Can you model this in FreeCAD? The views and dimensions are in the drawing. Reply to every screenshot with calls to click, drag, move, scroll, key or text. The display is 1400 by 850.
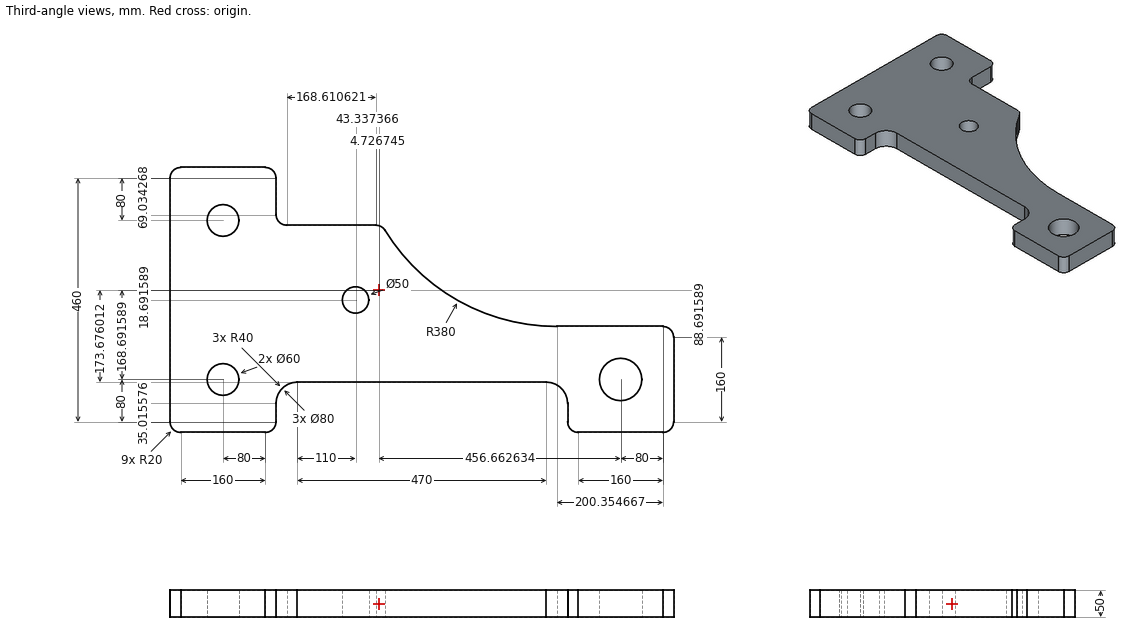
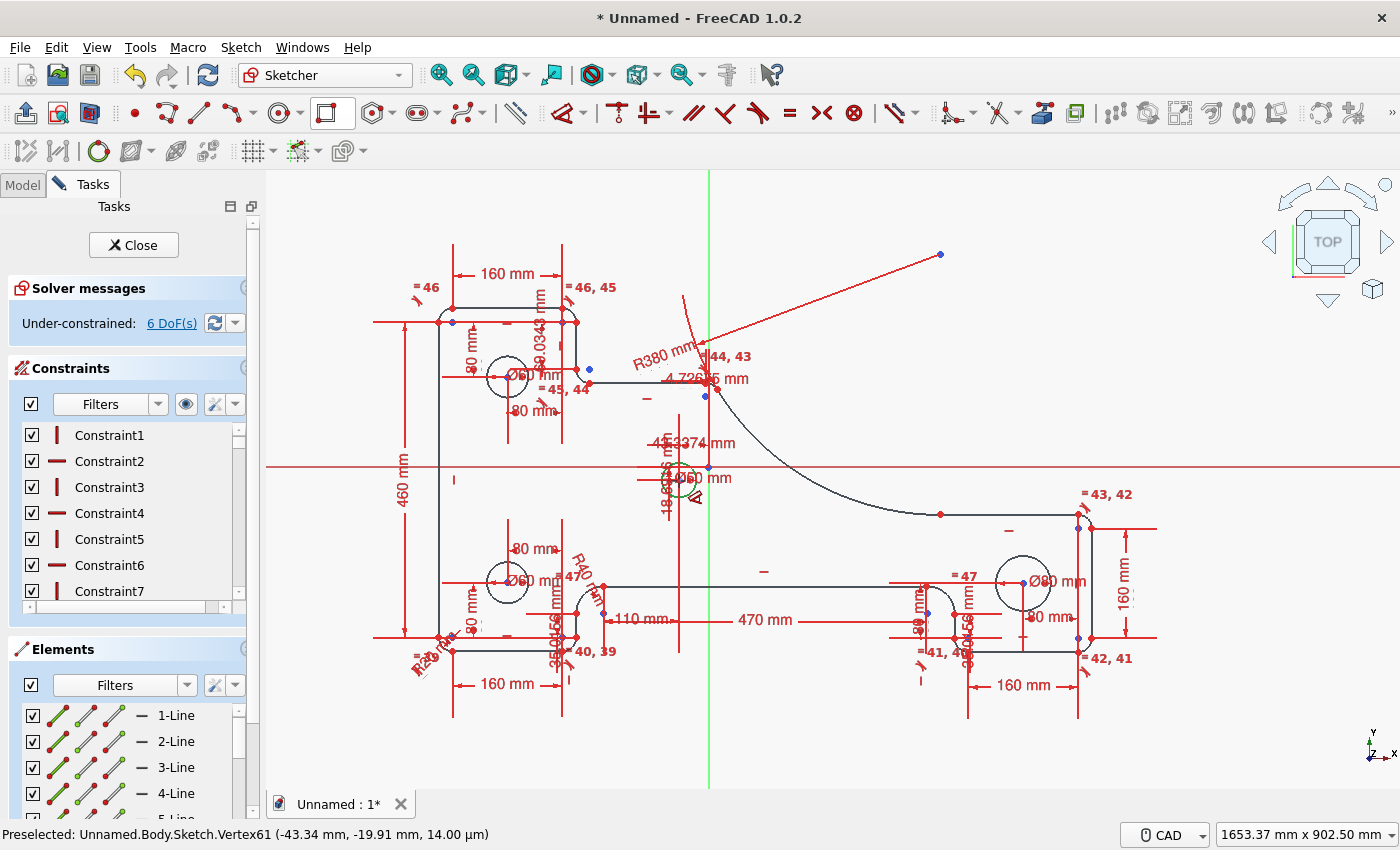
click(1037, 515)
click(977, 549)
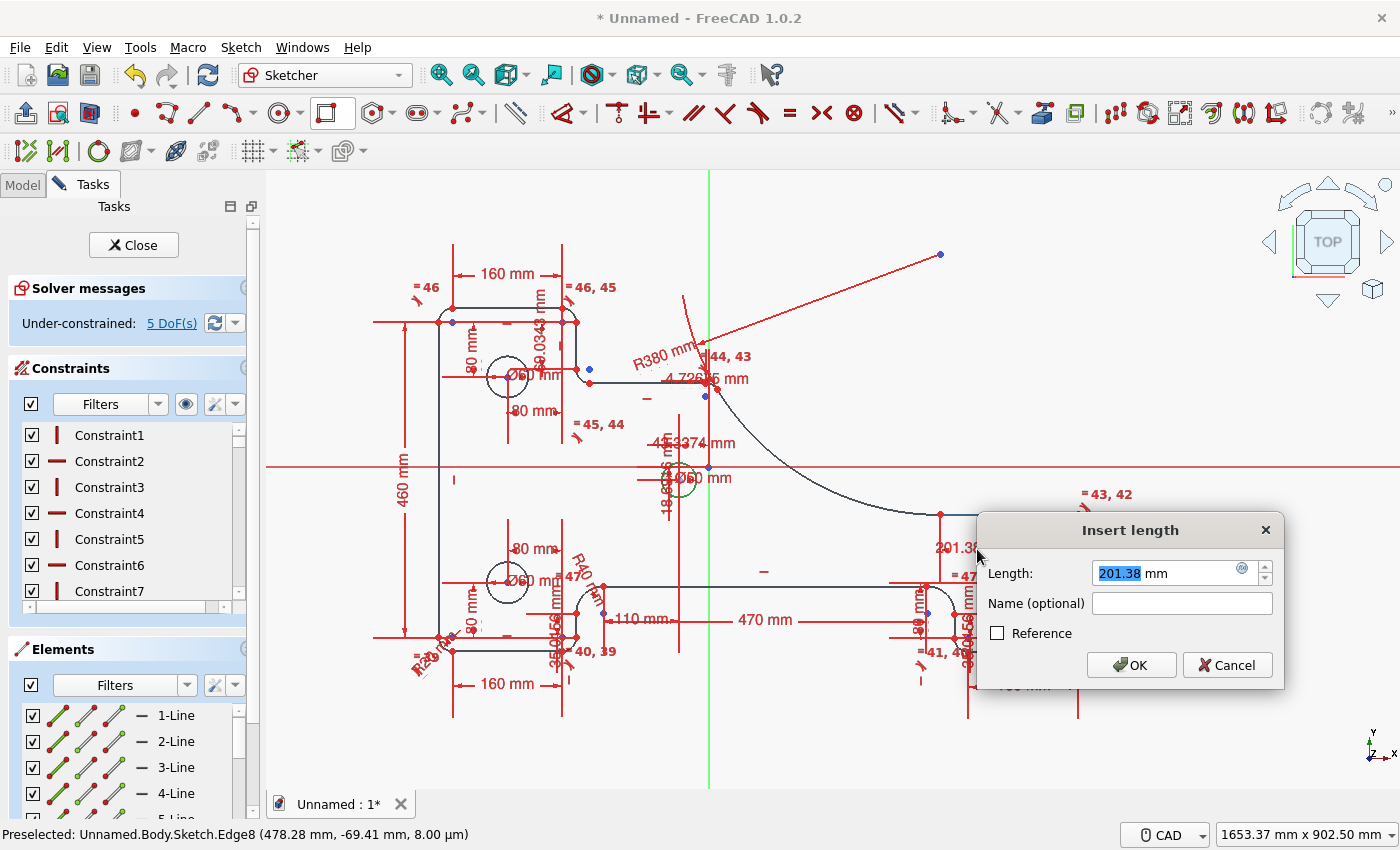
text(200.354667)
key(Return)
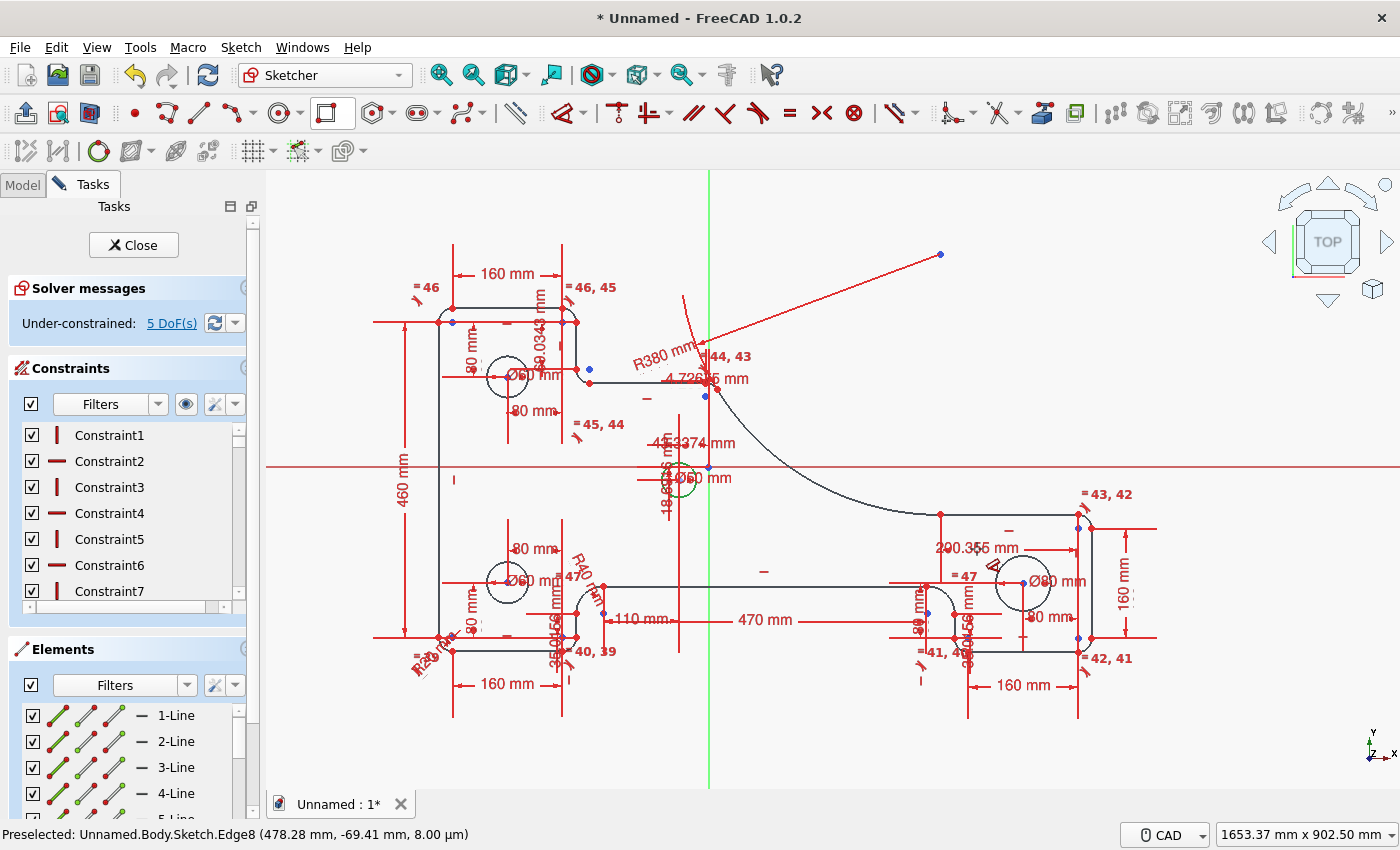
click(671, 383)
click(648, 417)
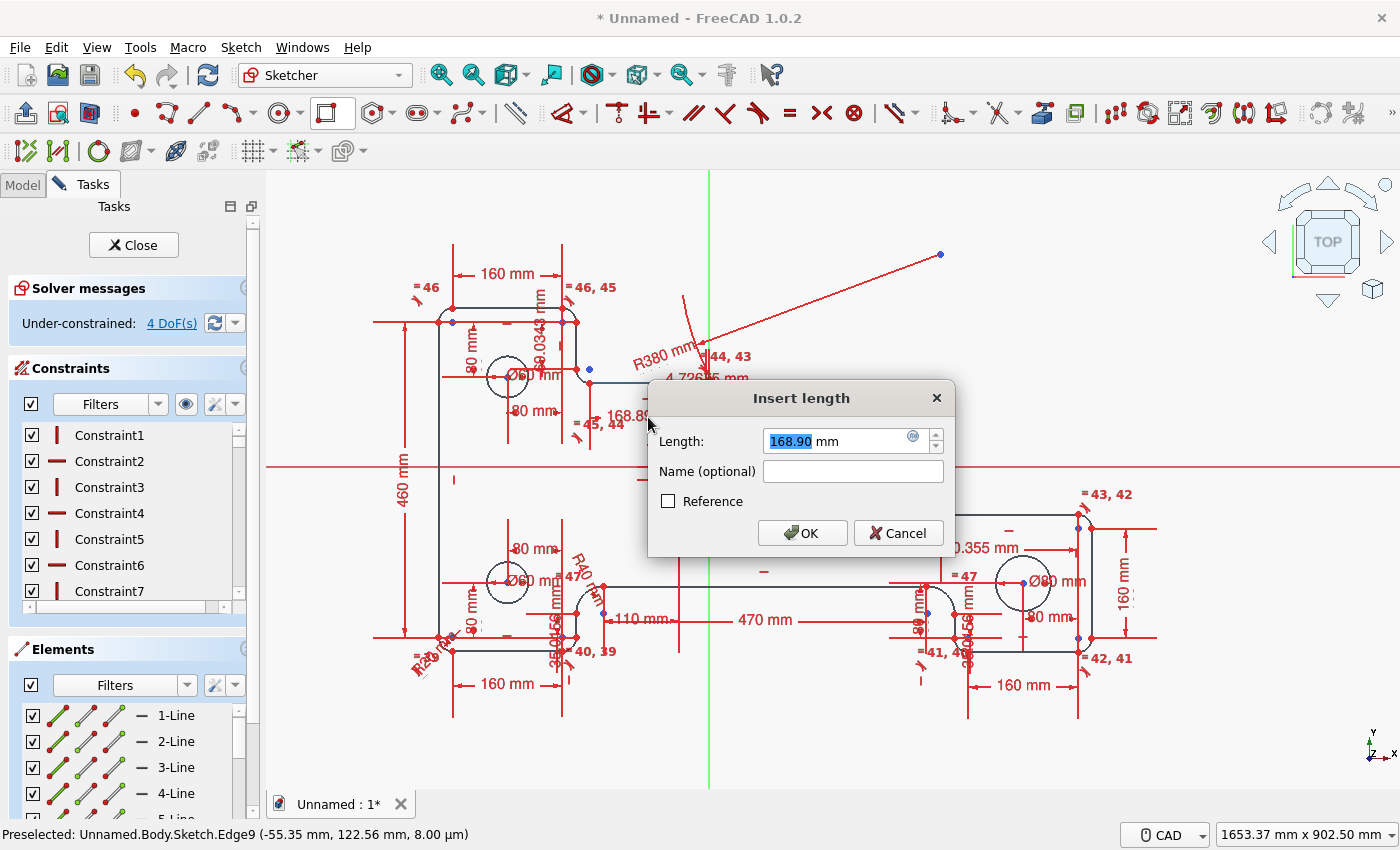
text(168.610621)
key(Return)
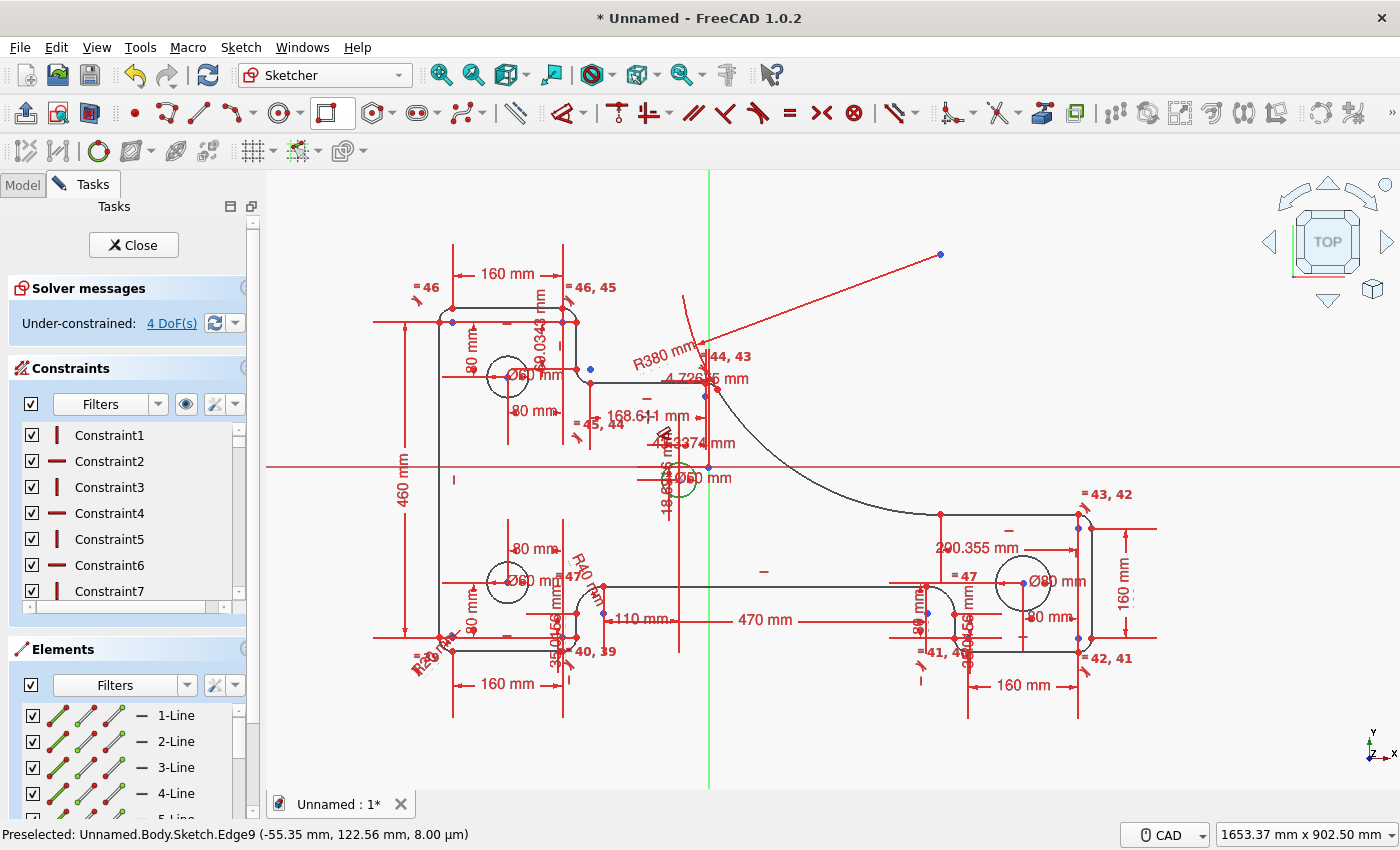
click(1092, 529)
click(1126, 498)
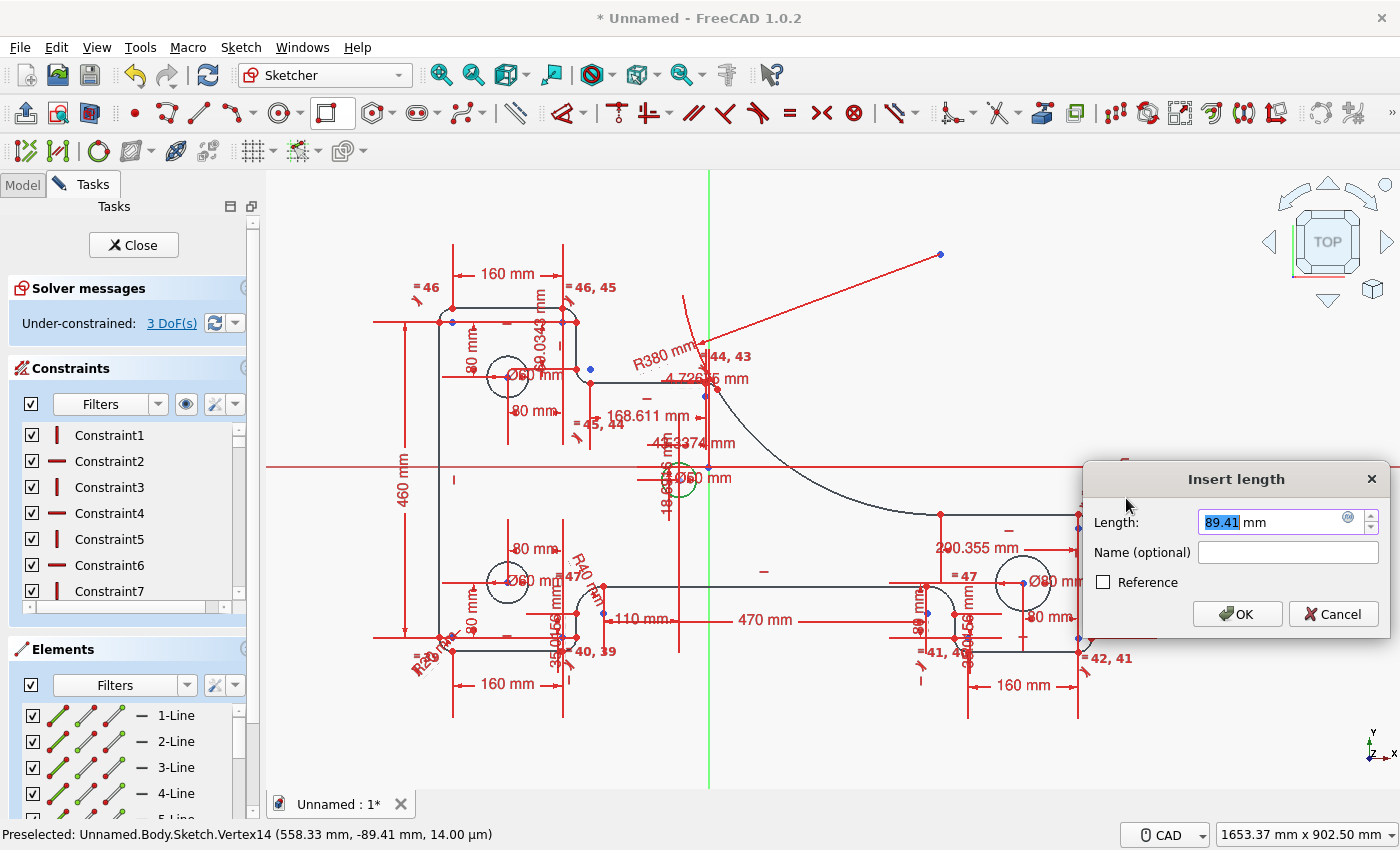
text(88.691589)
key(Return)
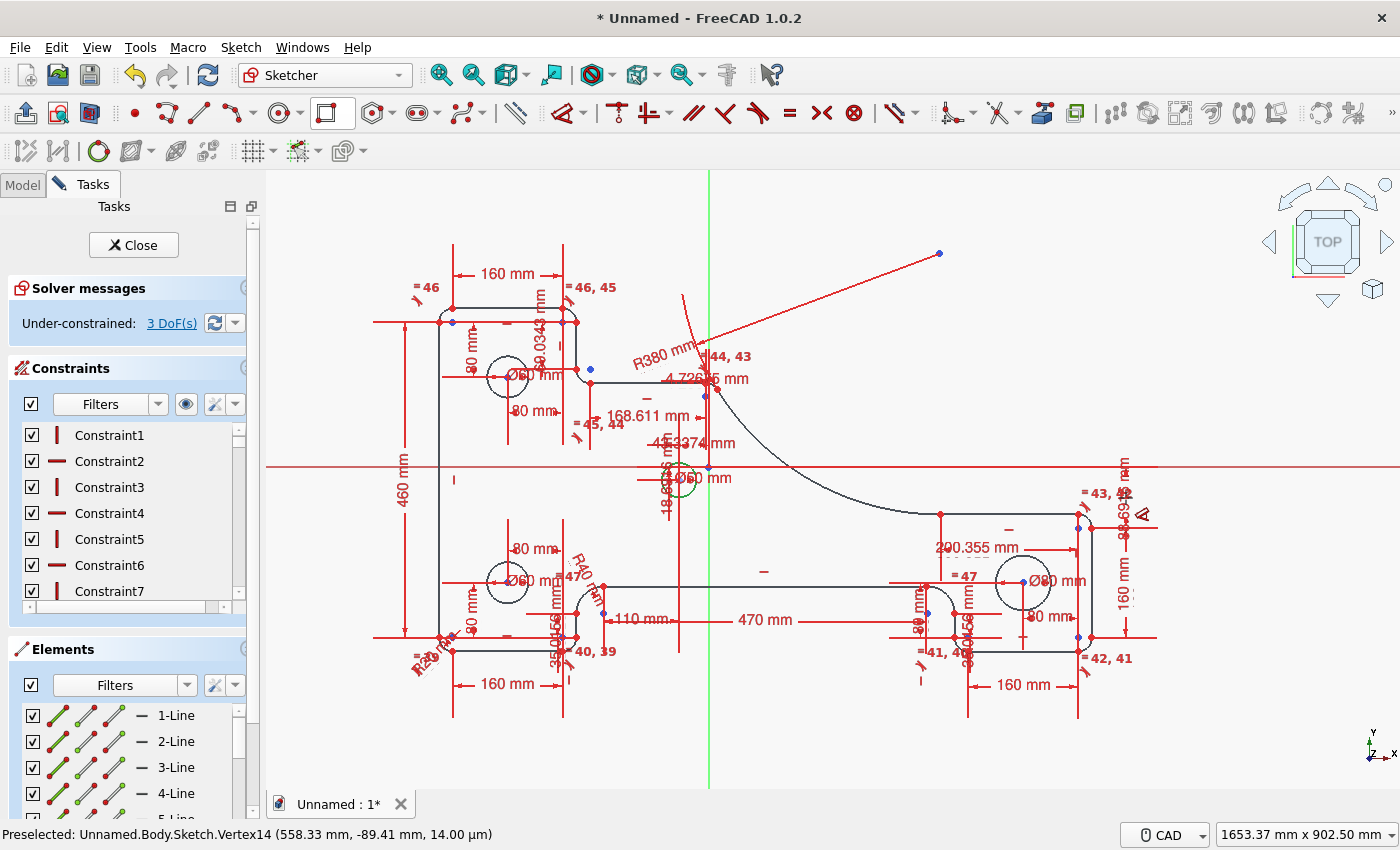
click(508, 583)
click(474, 525)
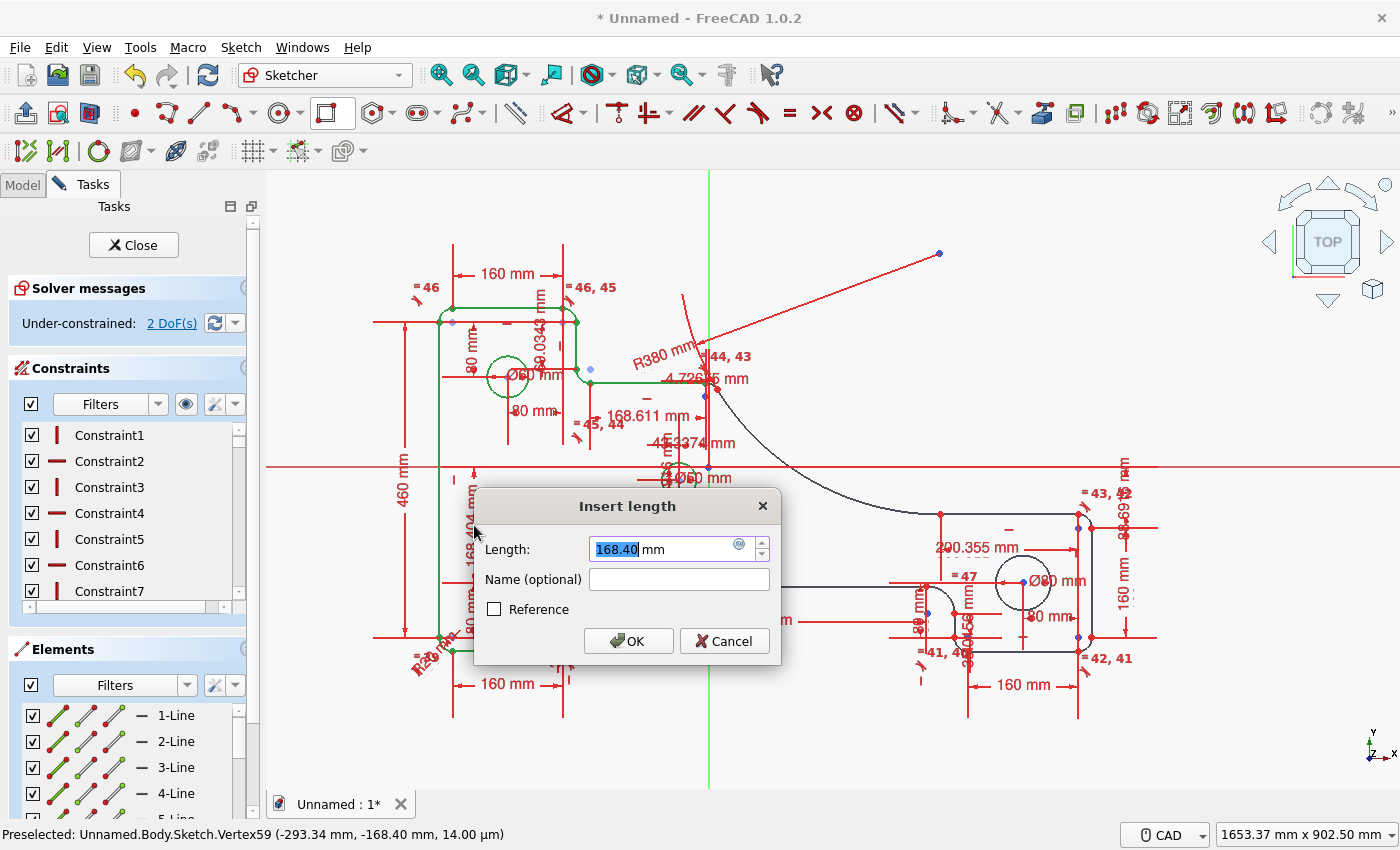
text(168.691589)
key(Return)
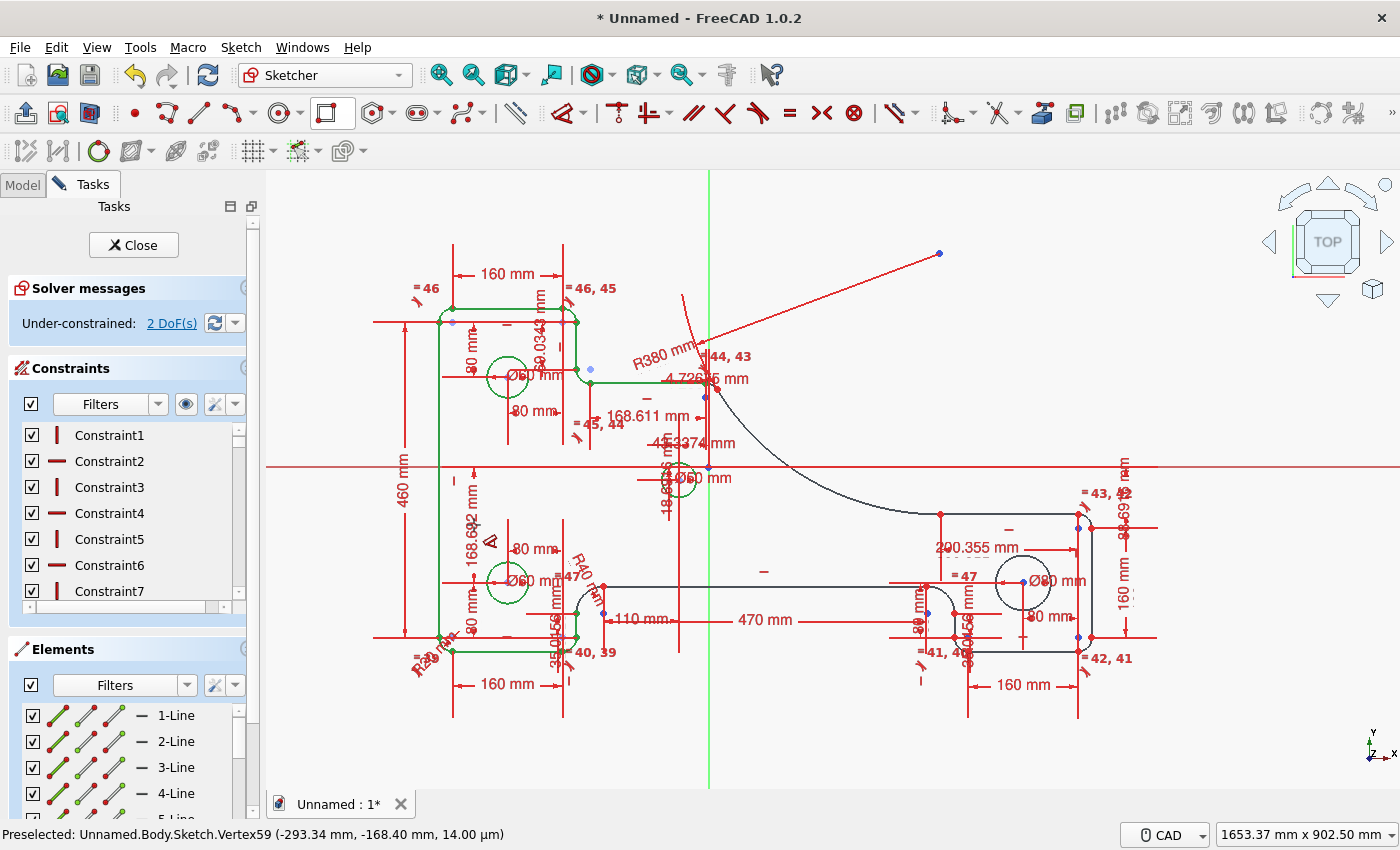
click(1023, 583)
click(866, 433)